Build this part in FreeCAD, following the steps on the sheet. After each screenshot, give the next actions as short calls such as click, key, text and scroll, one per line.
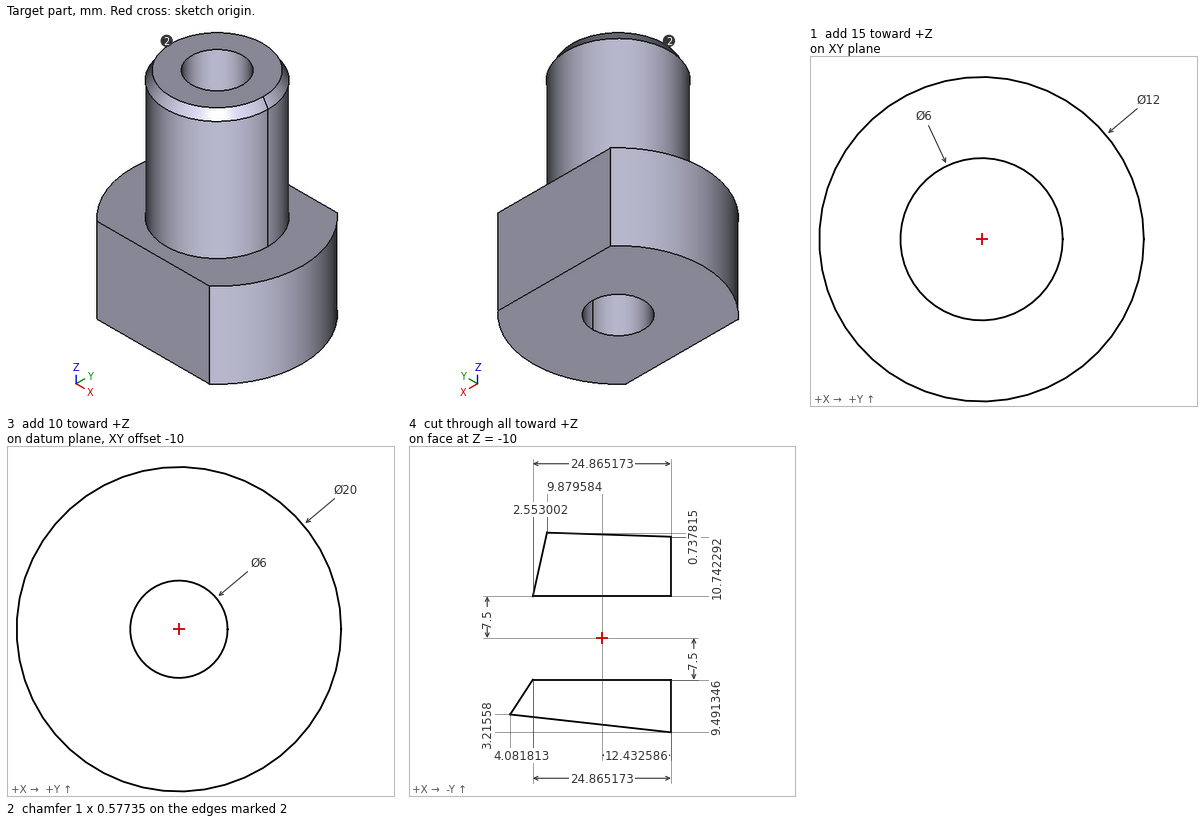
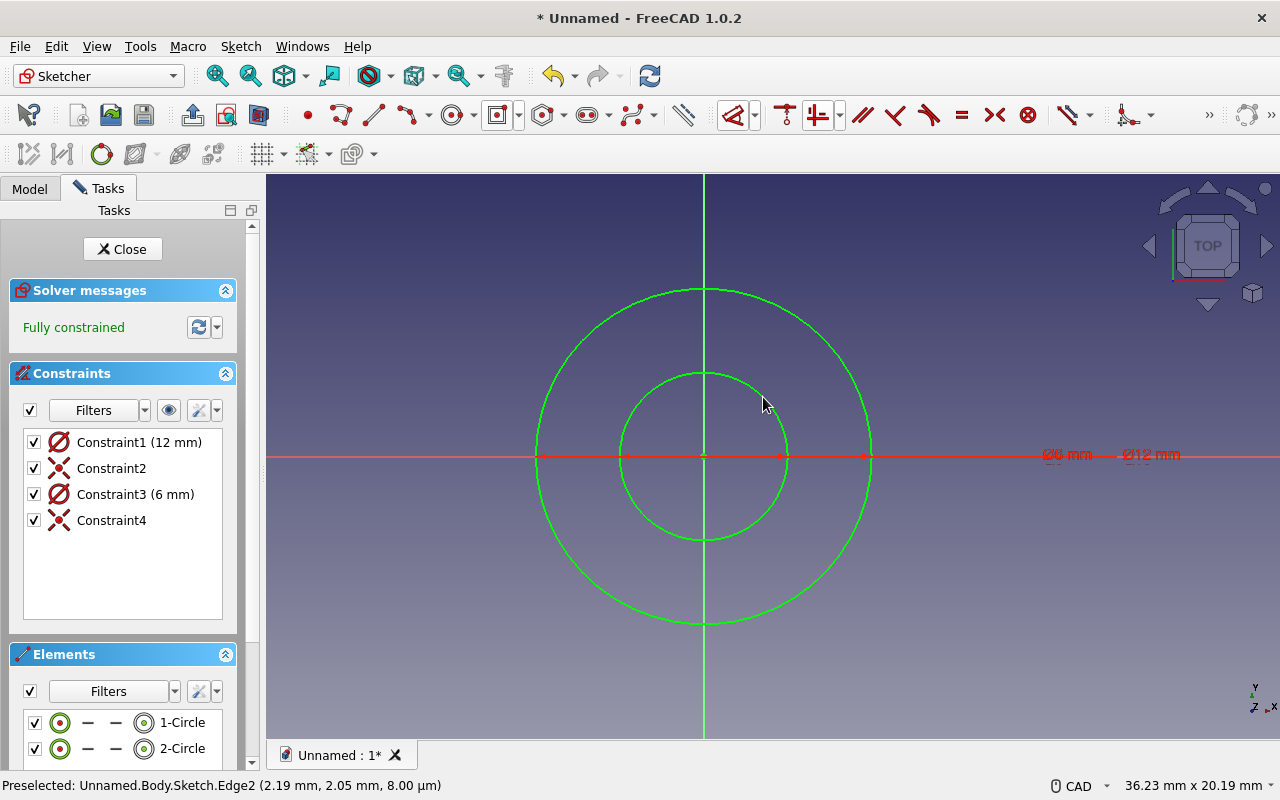
click(123, 249)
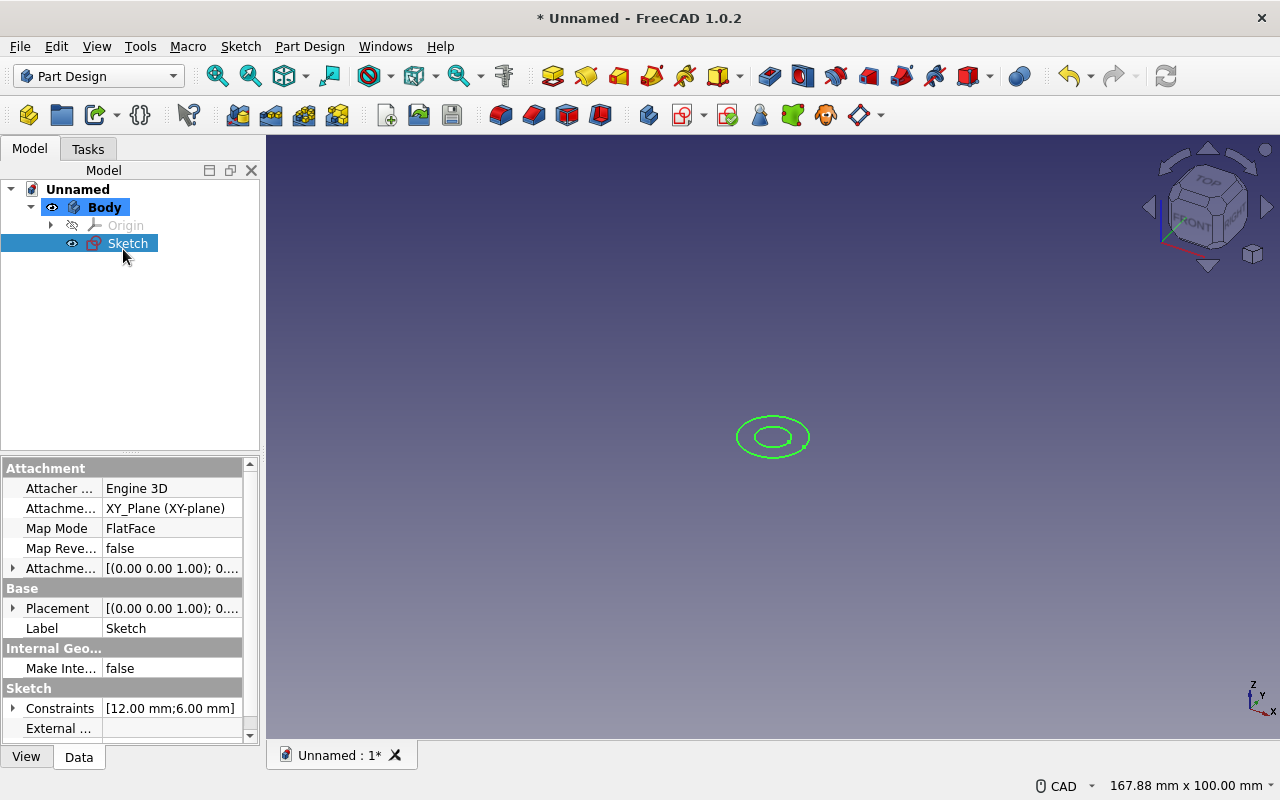
click(553, 76)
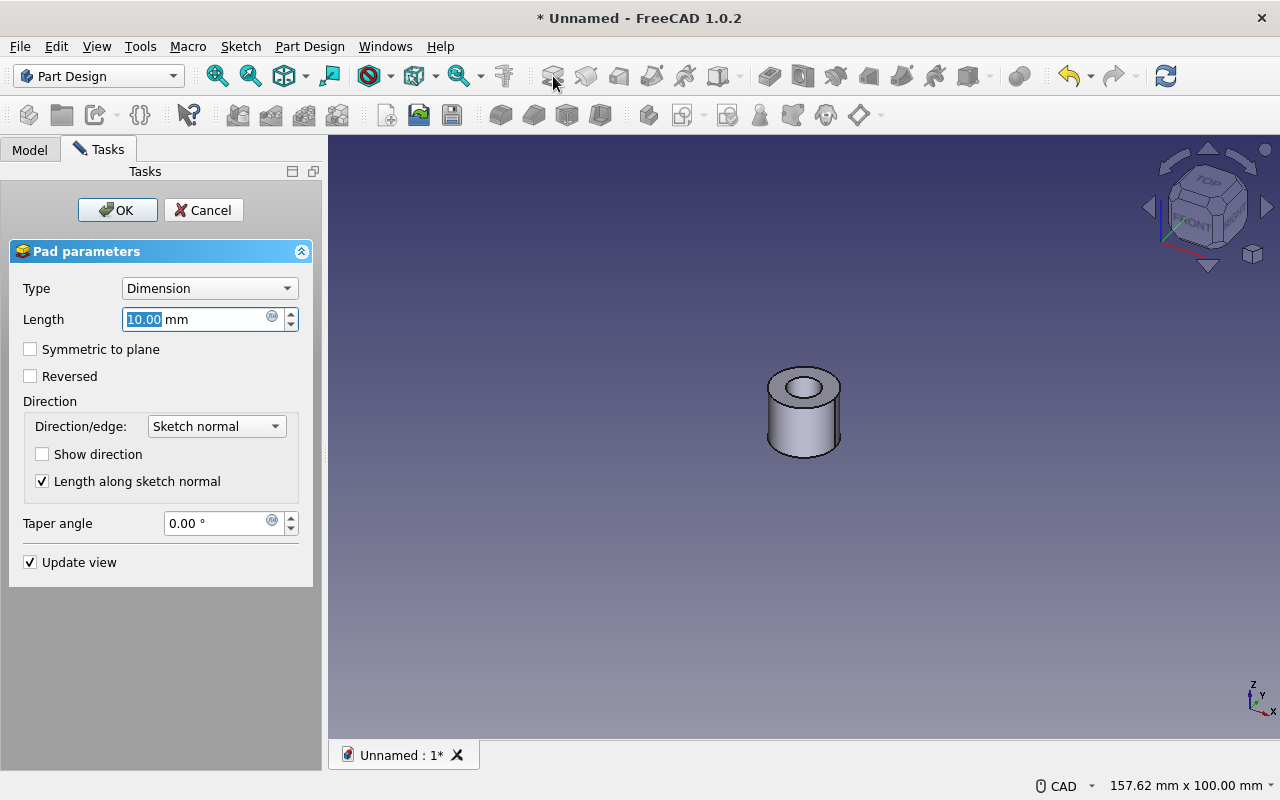
text(15)
key(Tab)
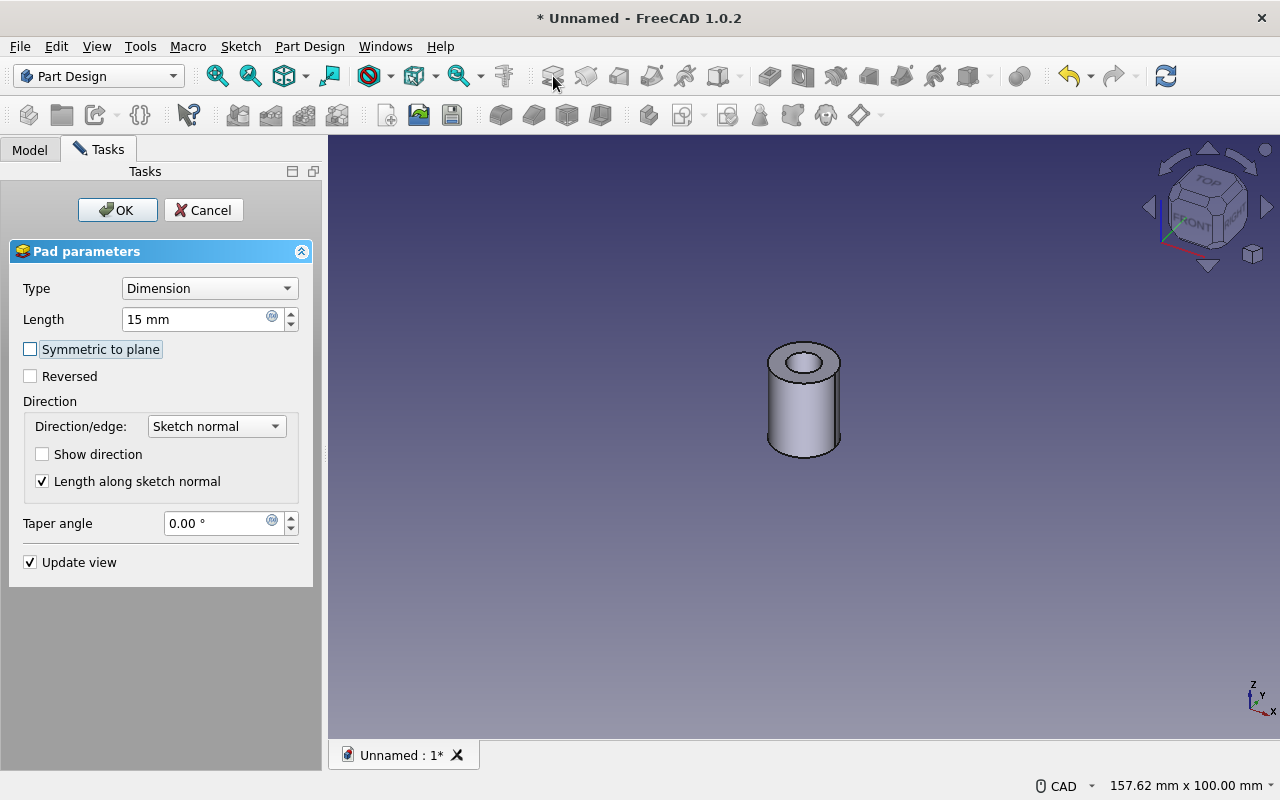
click(118, 210)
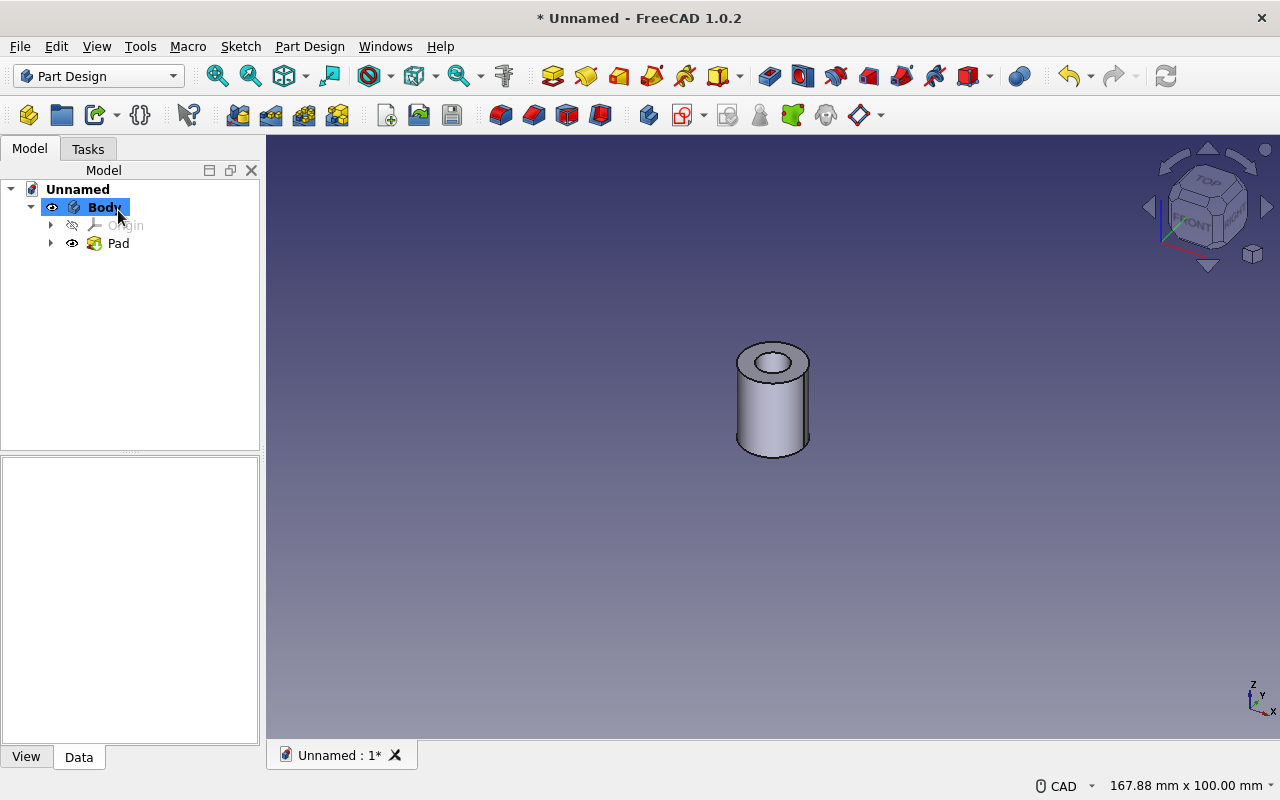
click(218, 76)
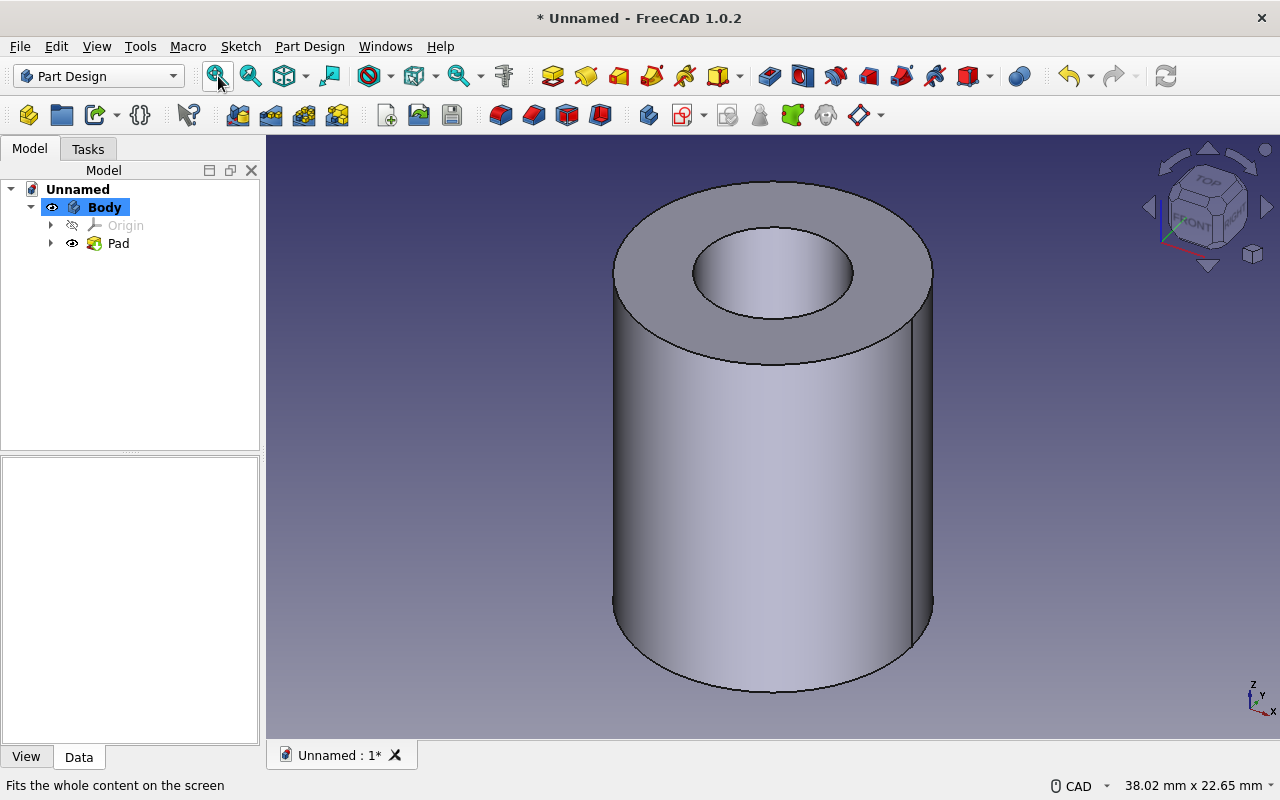
click(614, 282)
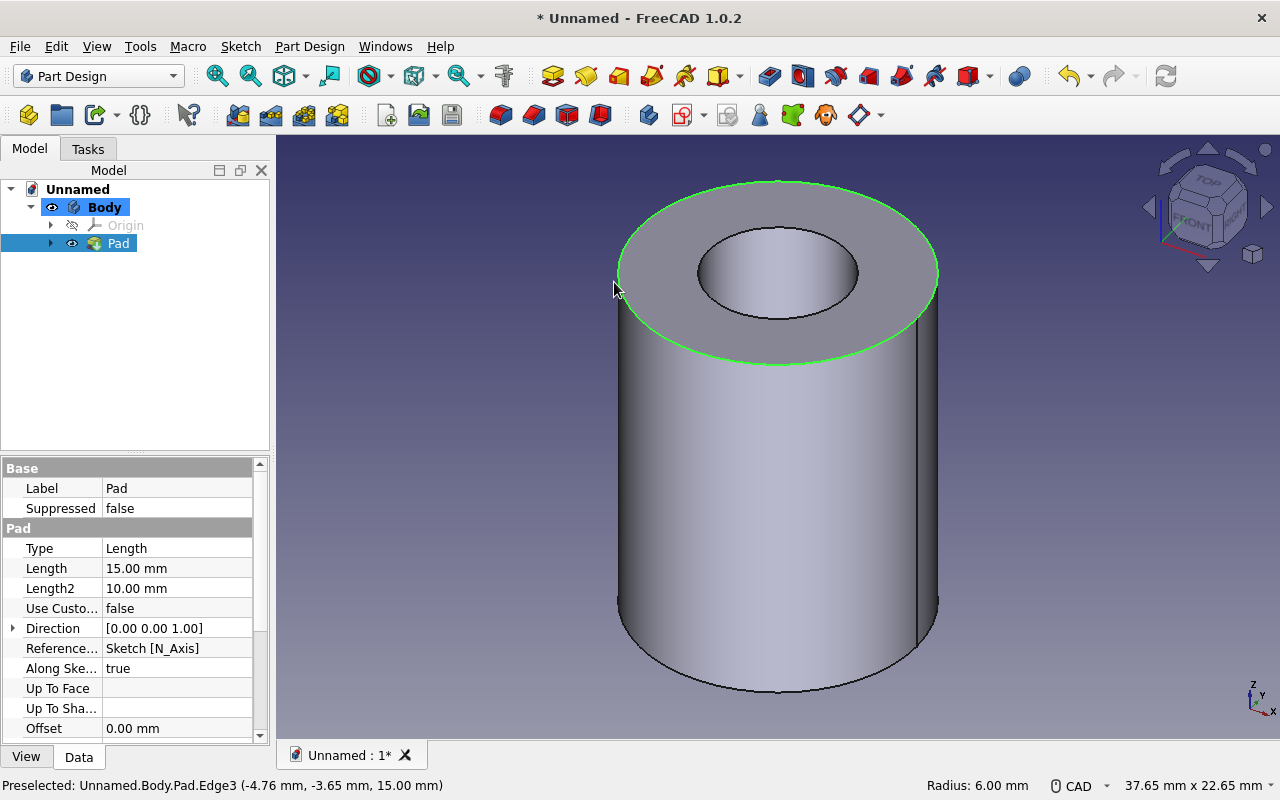
click(534, 116)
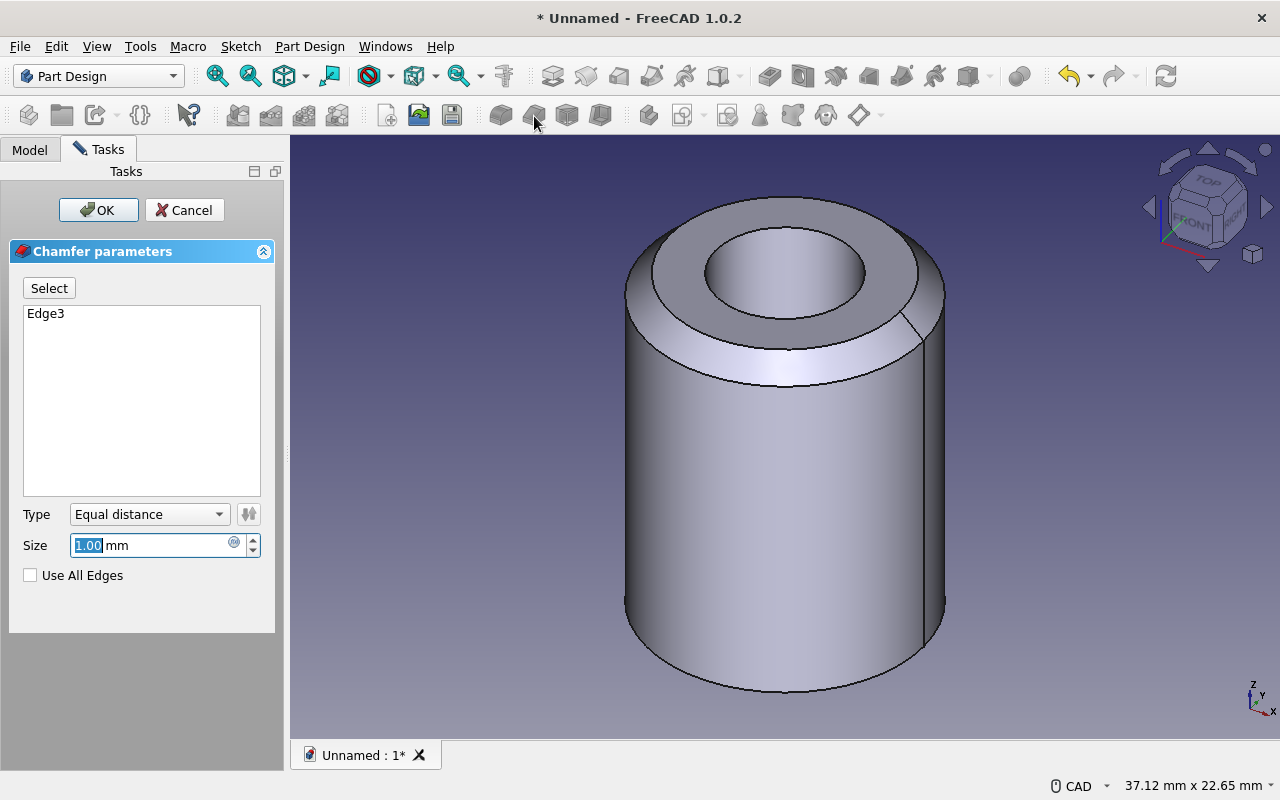
text(1)
key(Tab)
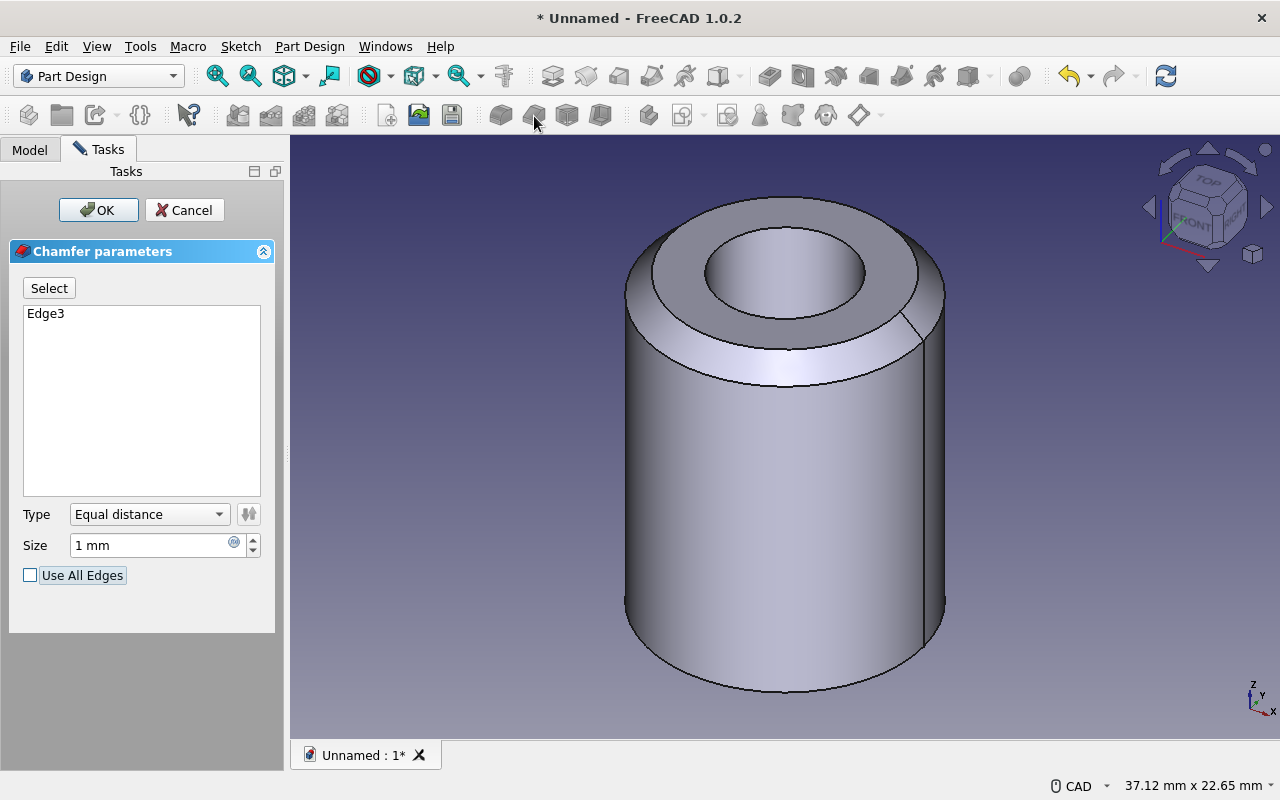
click(150, 514)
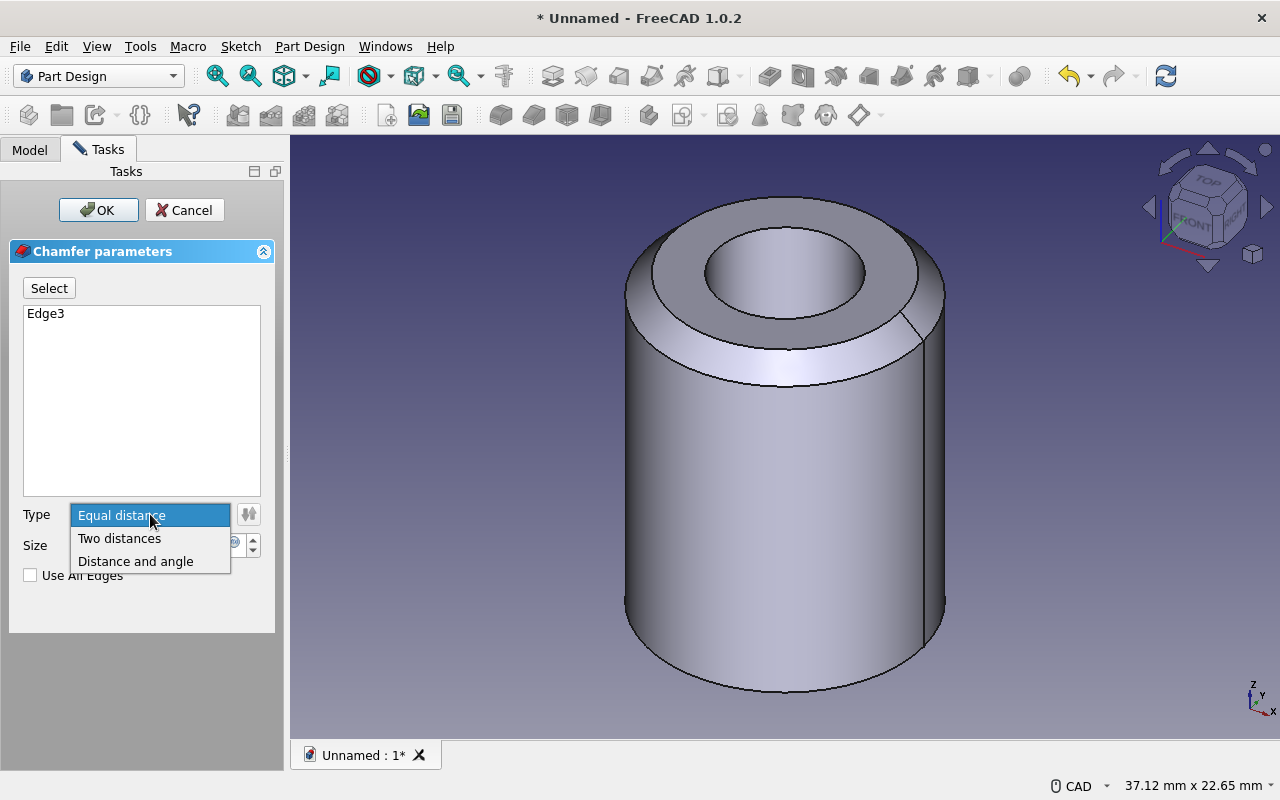
click(148, 538)